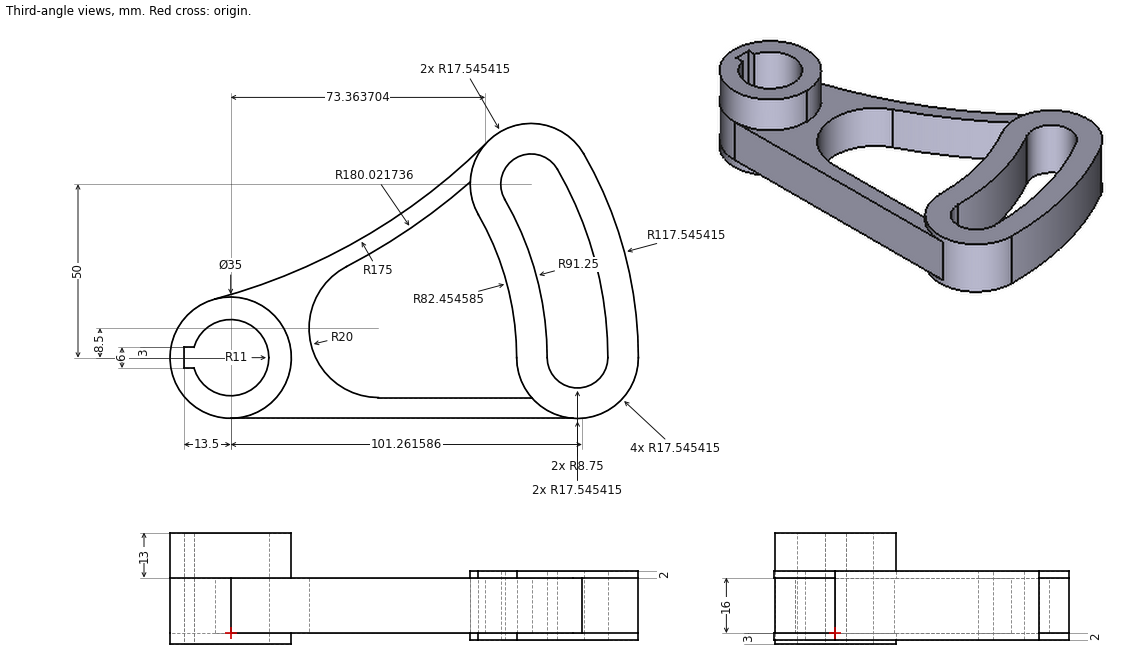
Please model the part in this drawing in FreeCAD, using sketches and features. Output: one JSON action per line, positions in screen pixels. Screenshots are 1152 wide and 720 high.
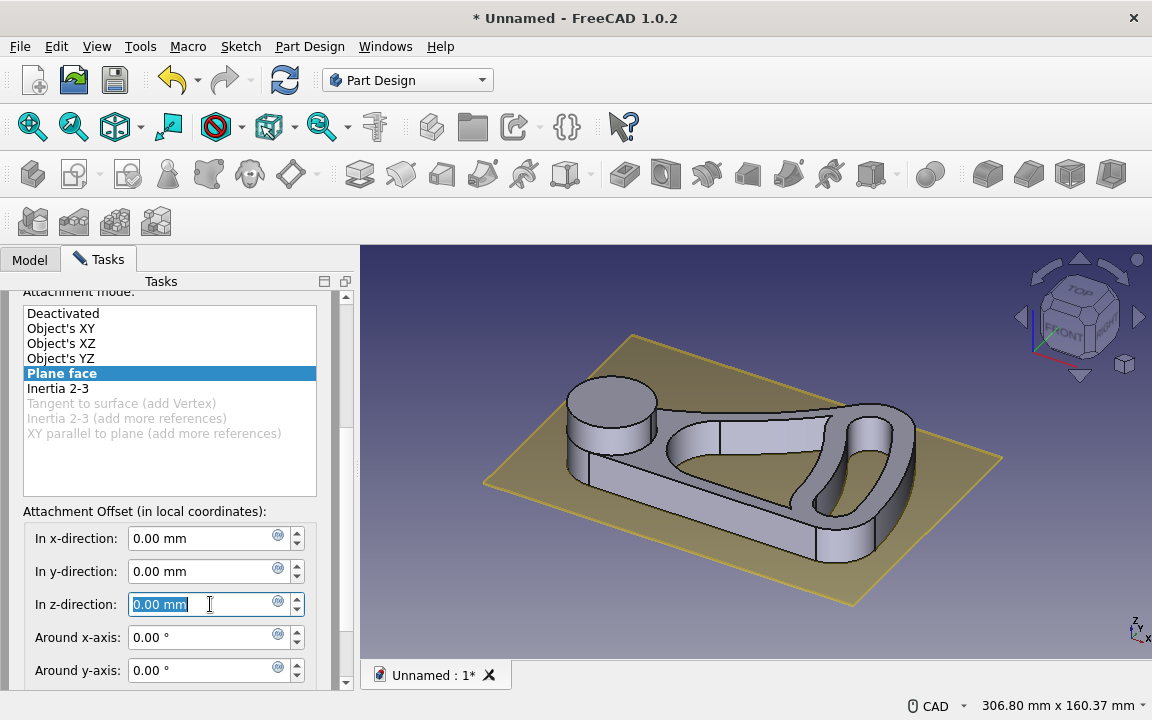
{"action": "type", "text": "-3"}
{"action": "key", "text": "Tab"}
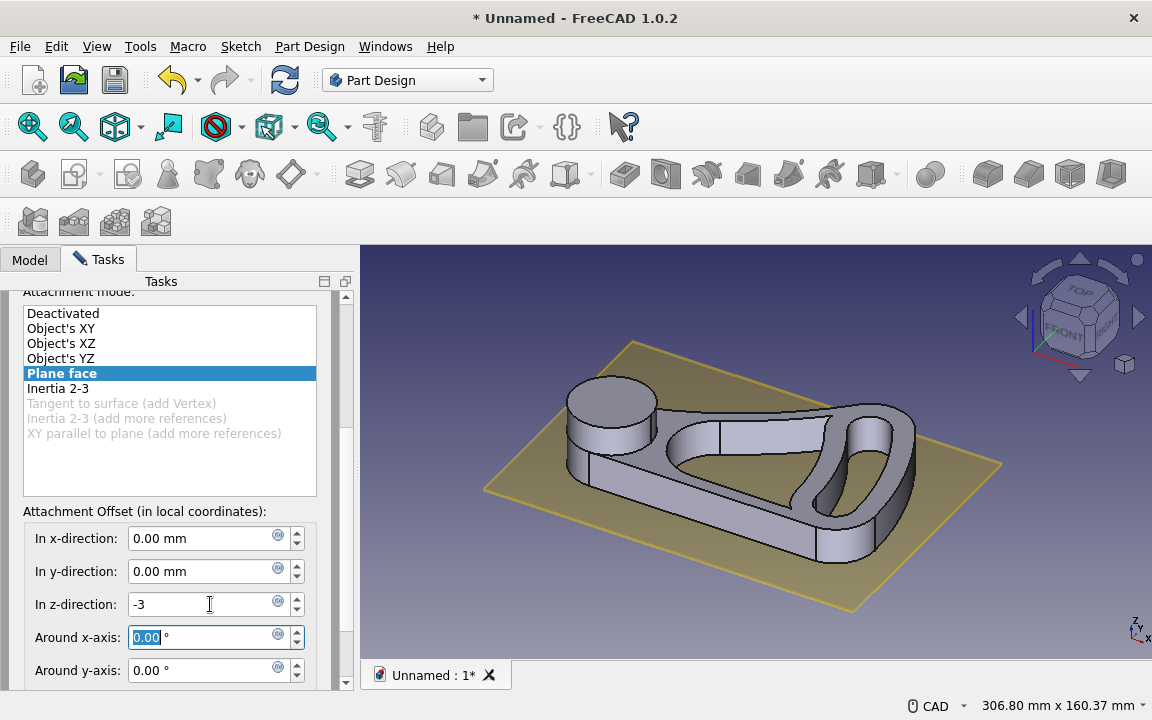
{"action": "scroll", "coordinate": [346, 490], "scroll_direction": "up", "scroll_amount": 5}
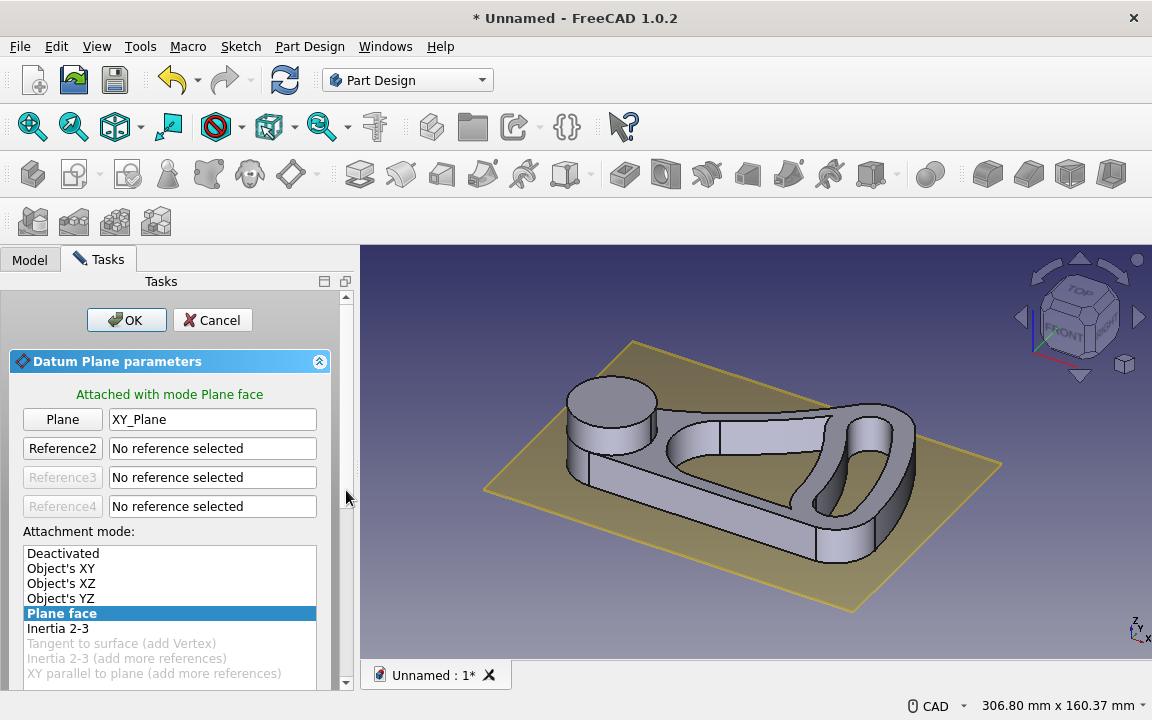
{"action": "left_click", "coordinate": [127, 320]}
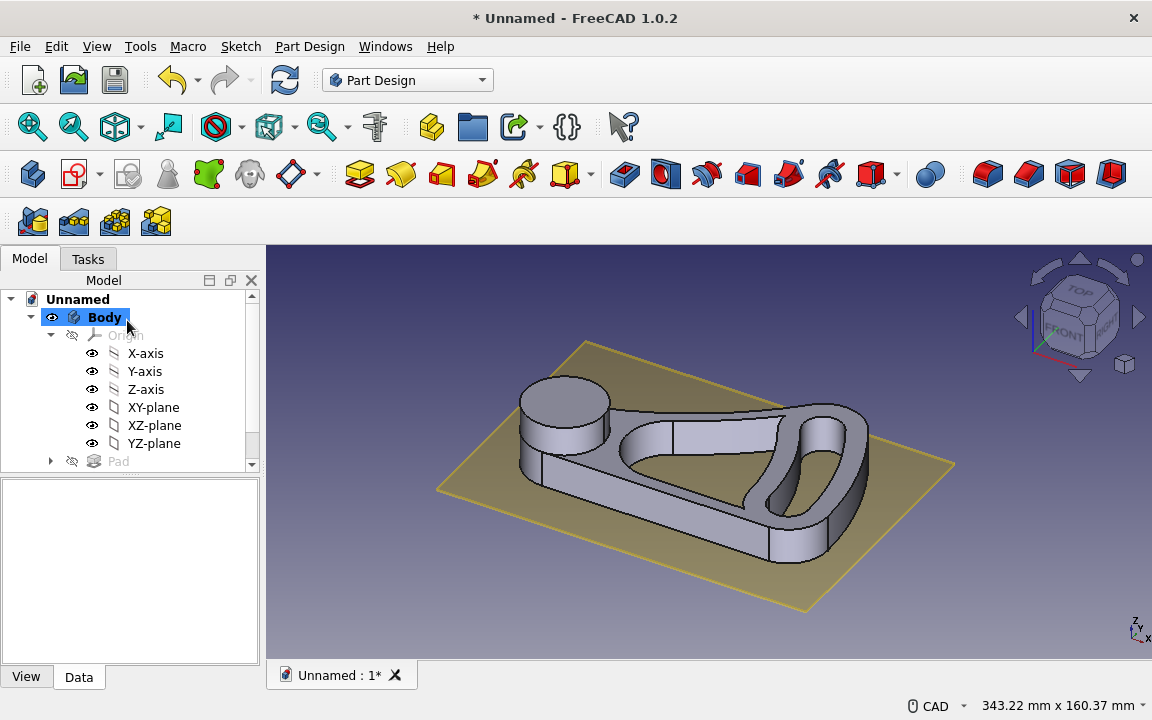
{"action": "scroll", "coordinate": [101, 385], "scroll_direction": "down", "scroll_amount": 3}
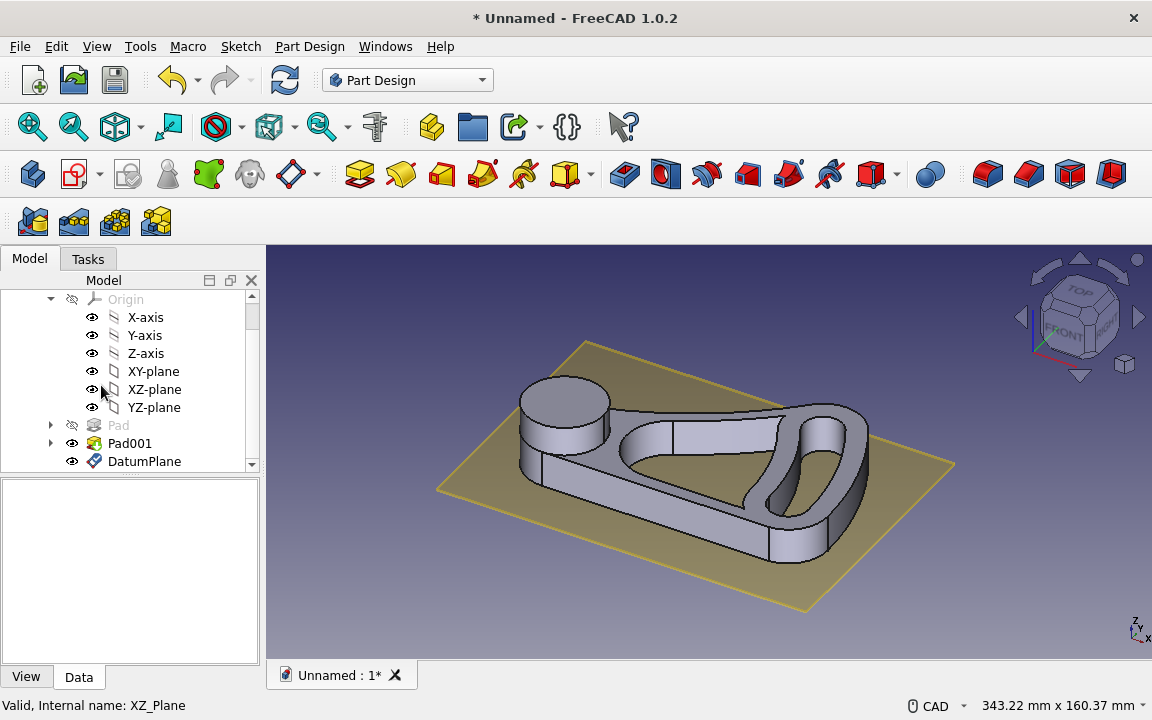
{"action": "left_click", "coordinate": [117, 461]}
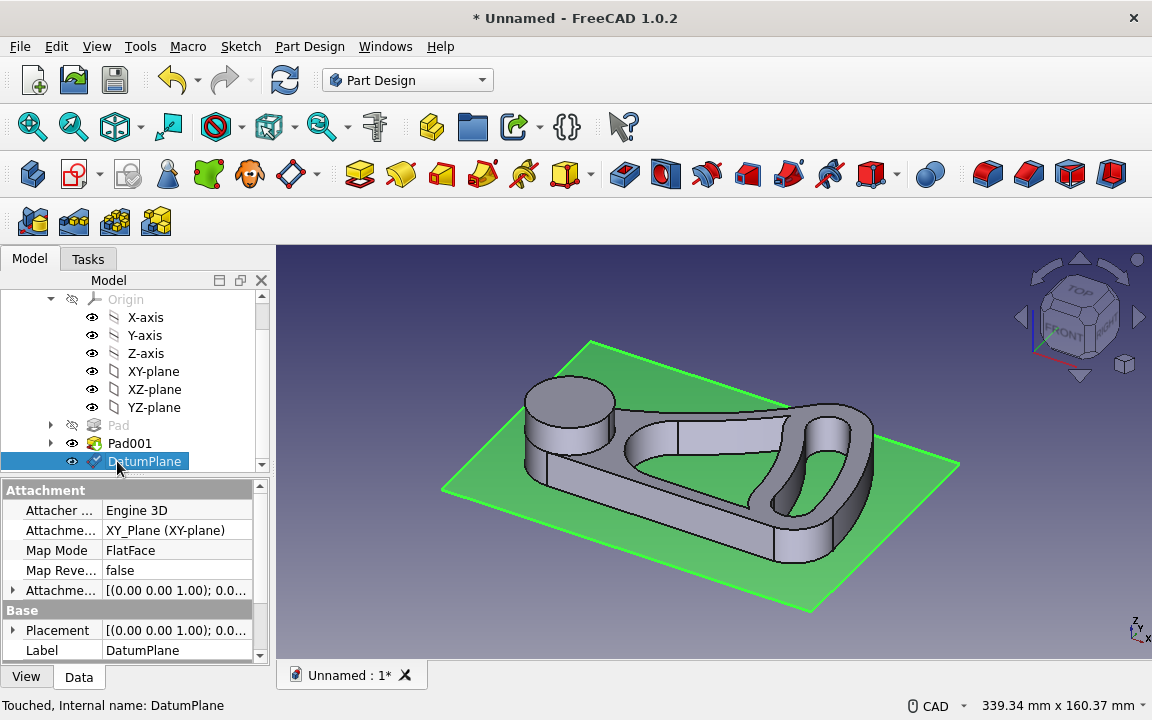
{"action": "left_click", "coordinate": [74, 174]}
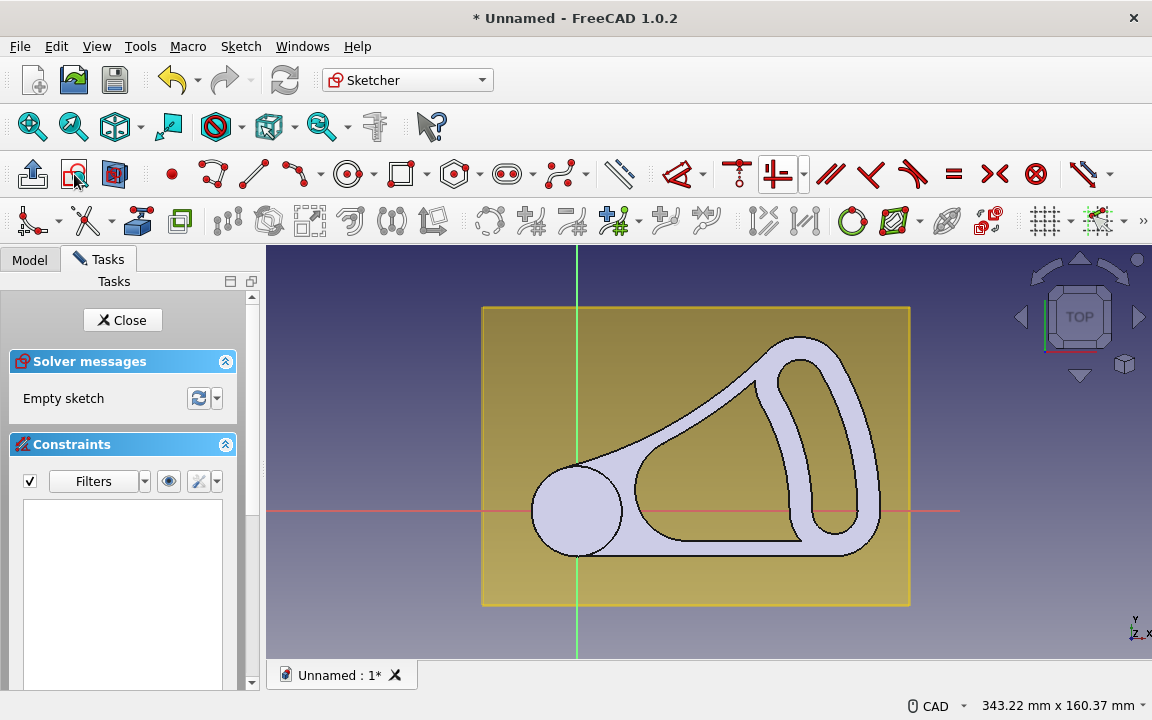
{"action": "left_click", "coordinate": [115, 174]}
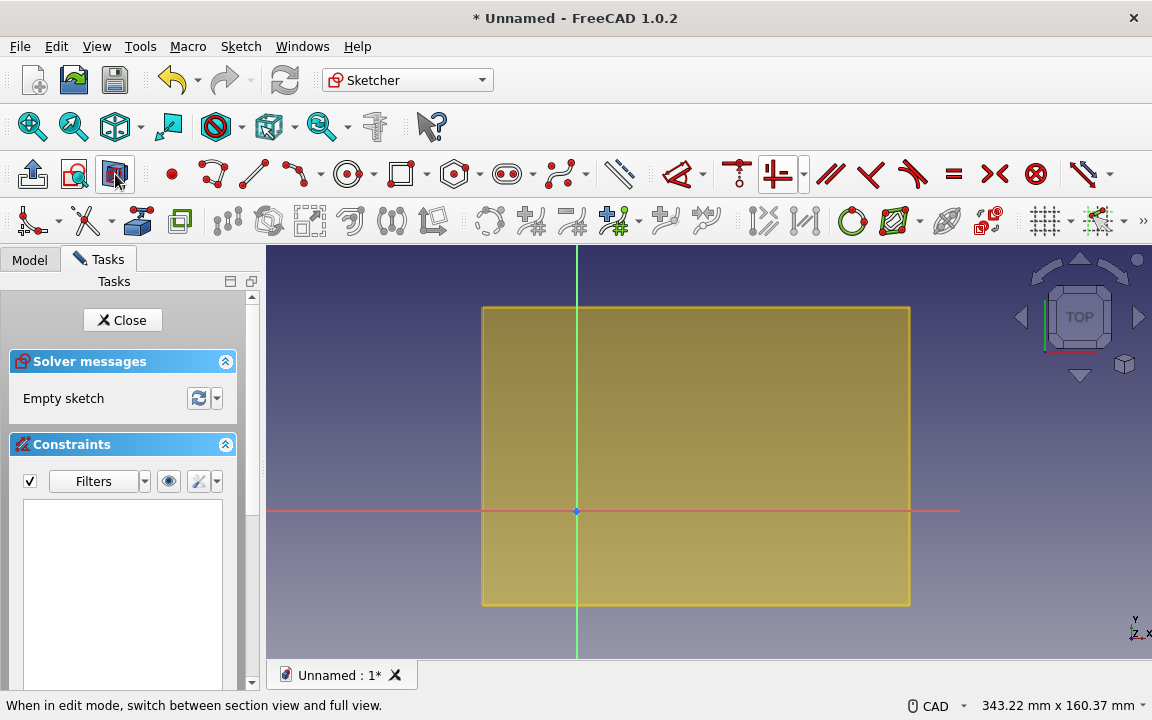
{"action": "scroll", "coordinate": [540, 546], "scroll_direction": "up", "scroll_amount": 5}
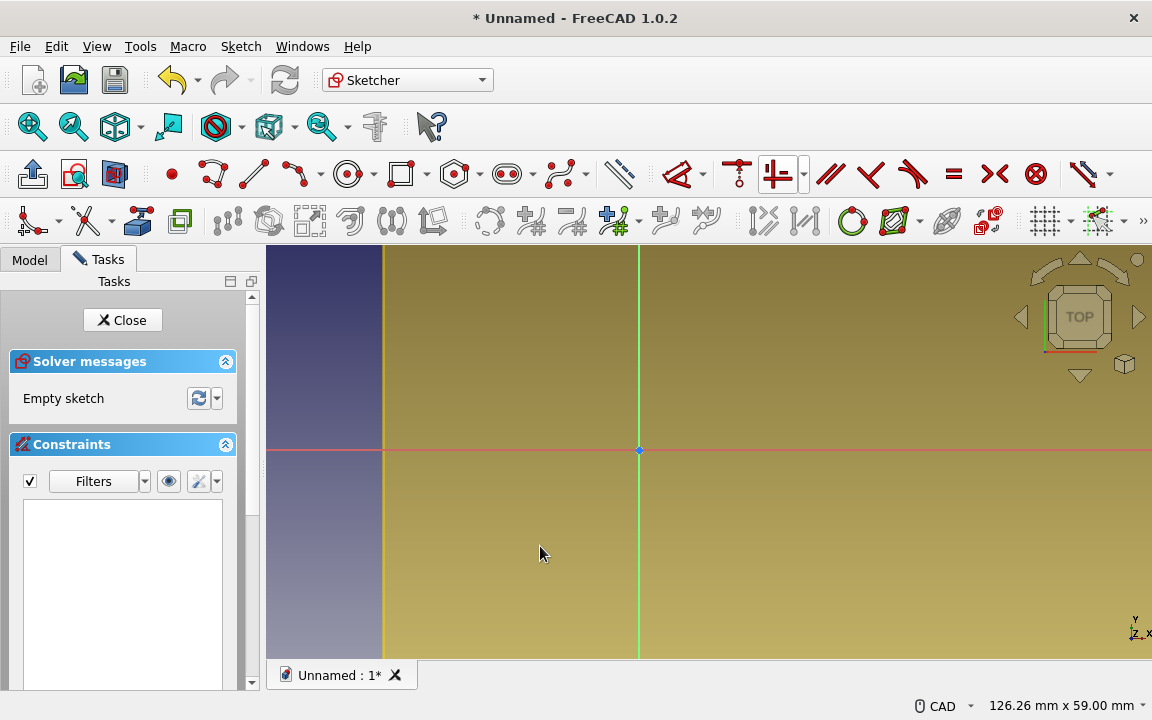
{"action": "left_click", "coordinate": [348, 174]}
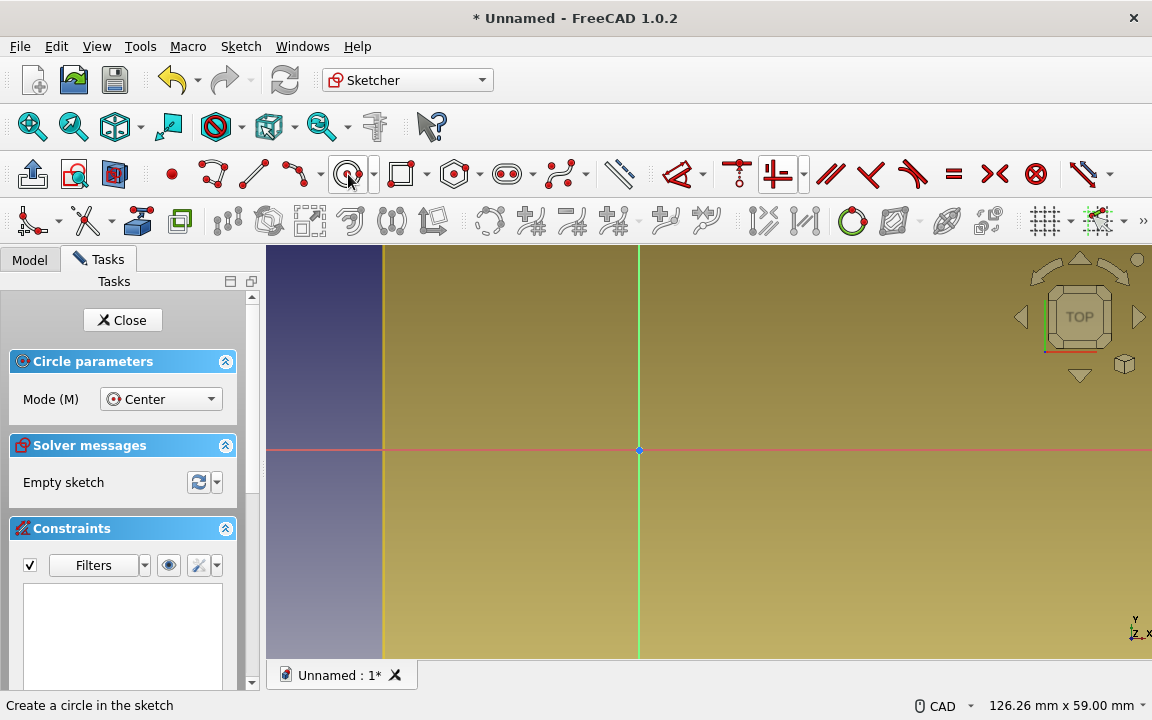
{"action": "left_click", "coordinate": [639, 450]}
{"action": "left_click", "coordinate": [726, 364]}
{"action": "key", "text": "Escape"}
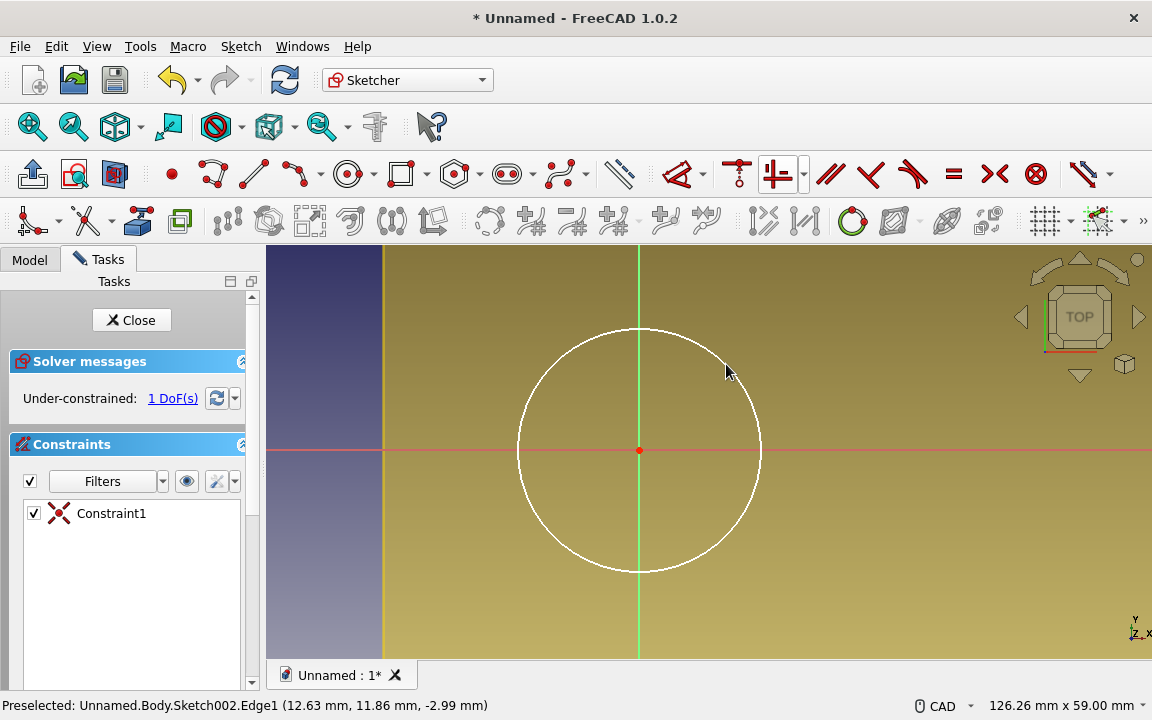
{"action": "left_click", "coordinate": [676, 174]}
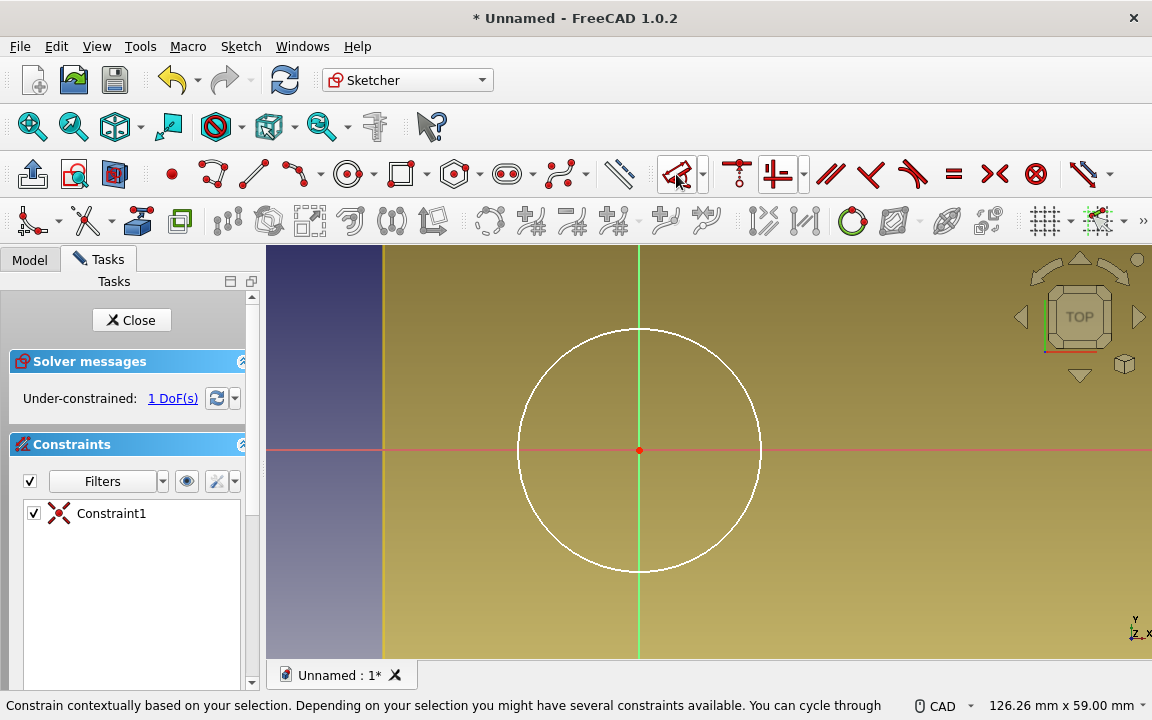
{"action": "left_click", "coordinate": [725, 364]}
{"action": "left_click", "coordinate": [747, 341]}